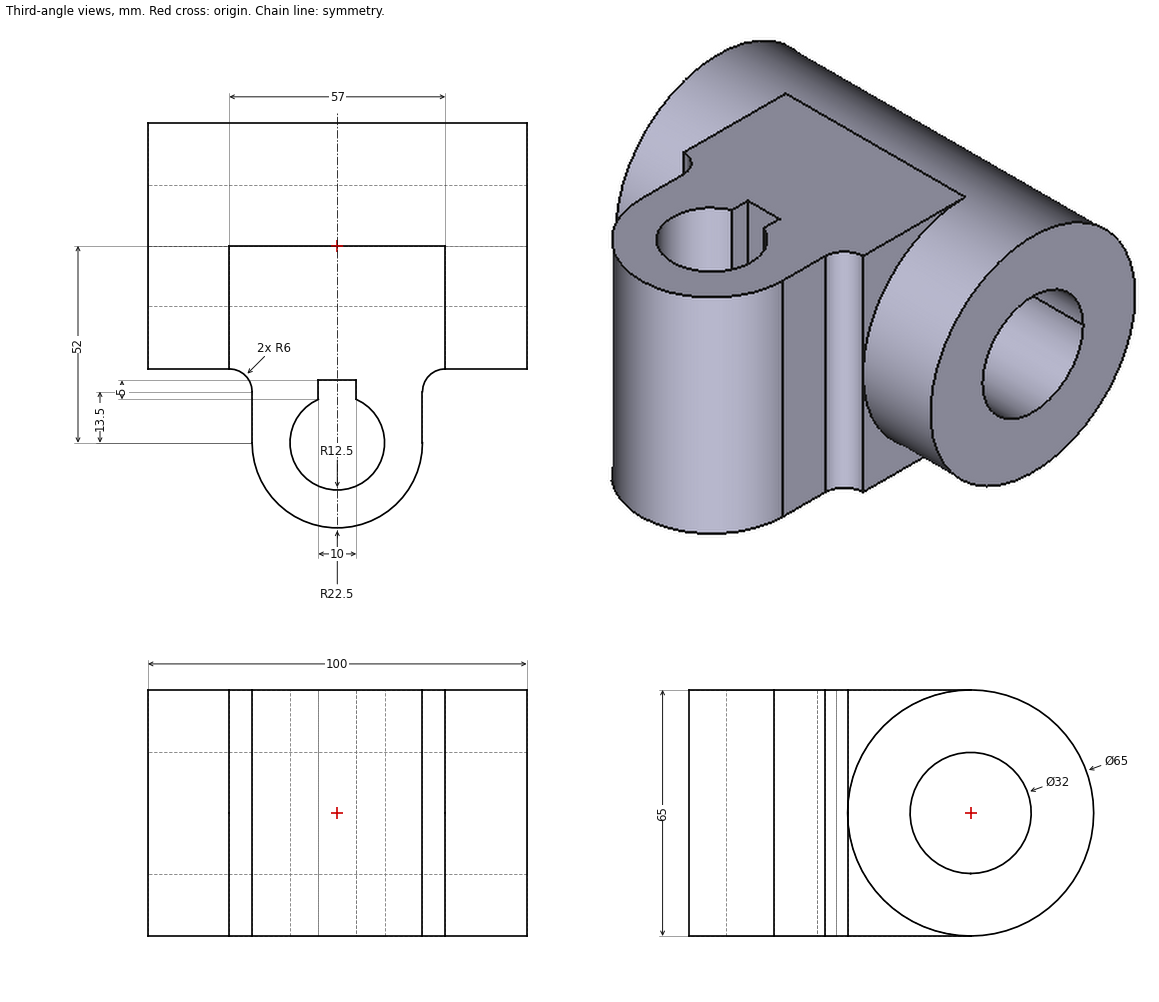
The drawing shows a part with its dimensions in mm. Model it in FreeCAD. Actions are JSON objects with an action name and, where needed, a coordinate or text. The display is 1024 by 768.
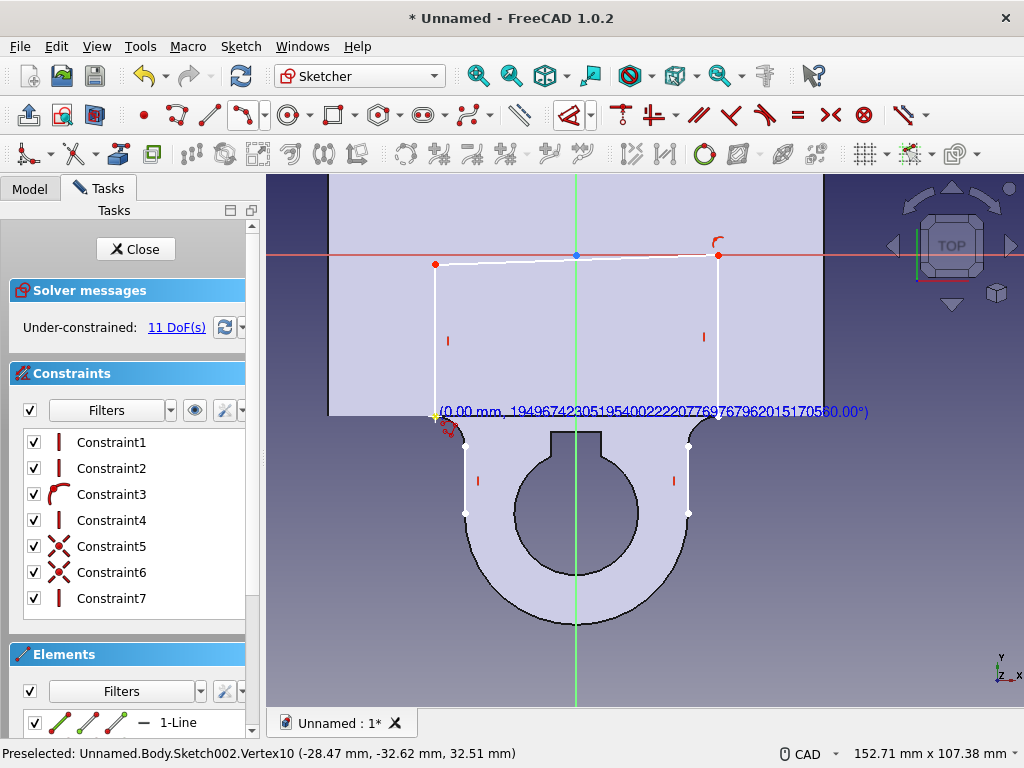
{"action": "left_click", "coordinate": [242, 116]}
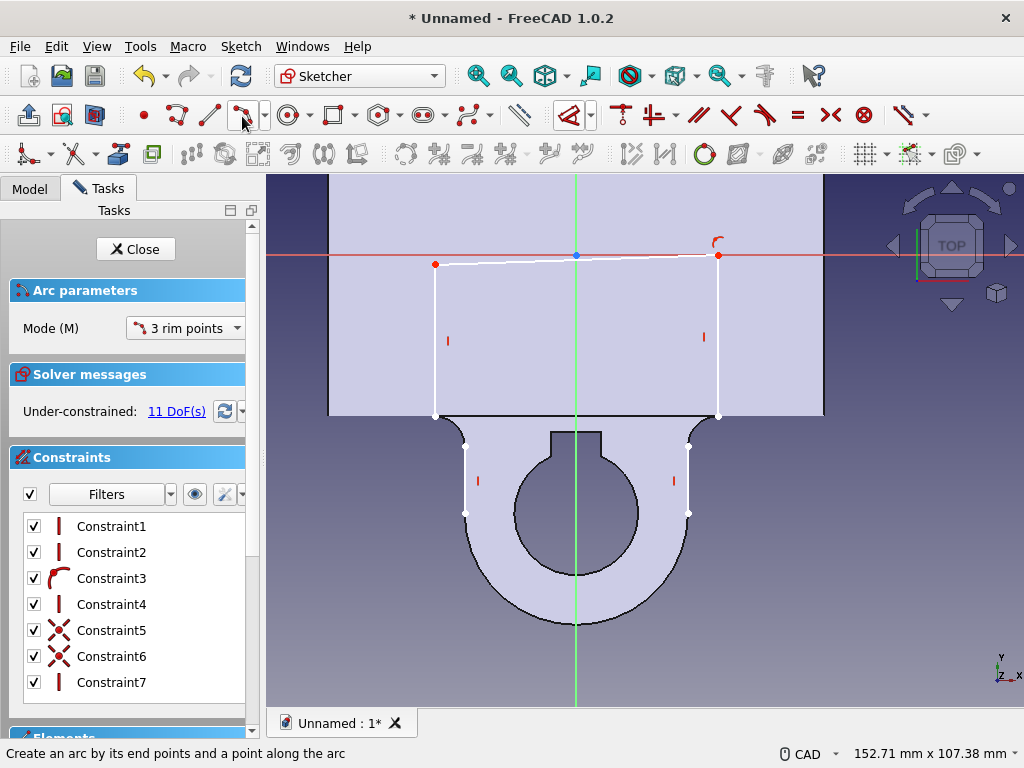
{"action": "left_click", "coordinate": [465, 514]}
{"action": "left_click", "coordinate": [688, 514]}
{"action": "left_click", "coordinate": [542, 619]}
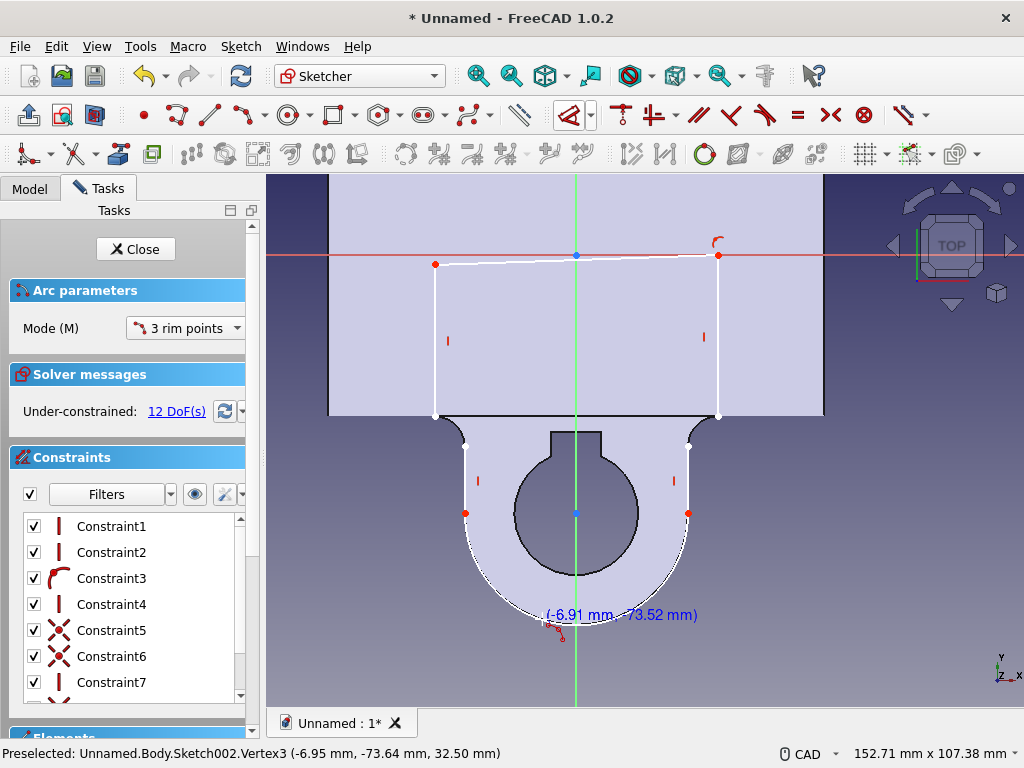
{"action": "left_click", "coordinate": [688, 447]}
{"action": "left_click", "coordinate": [718, 417]}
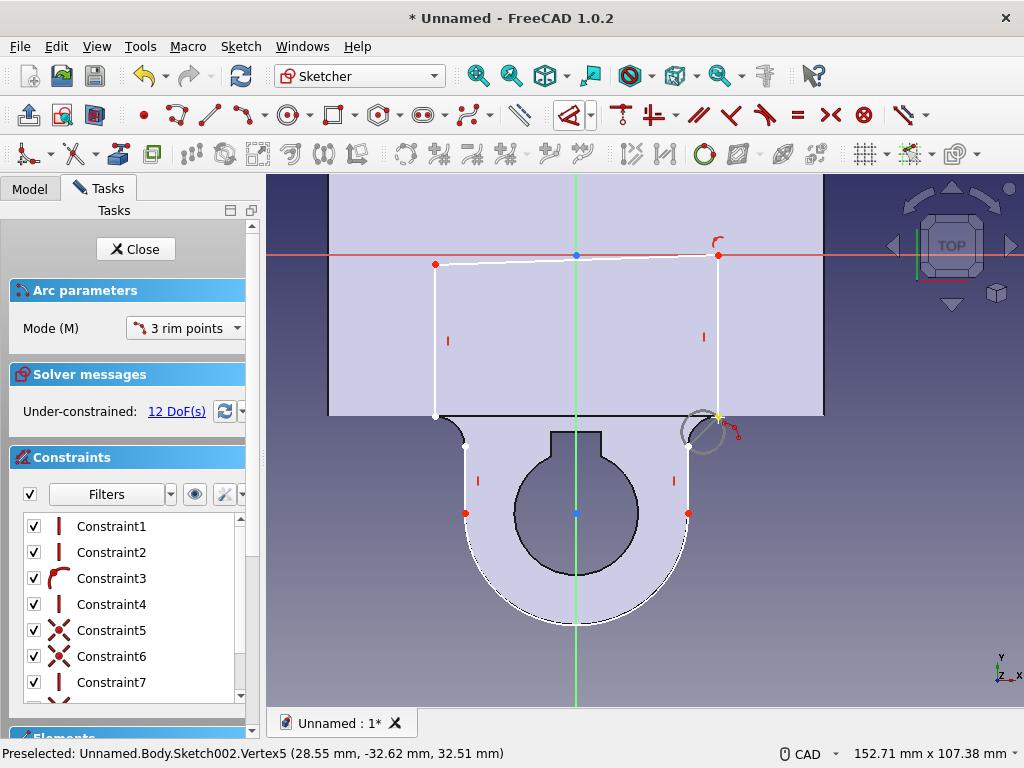
{"action": "scroll", "coordinate": [697, 425], "scroll_direction": "up", "scroll_amount": 3}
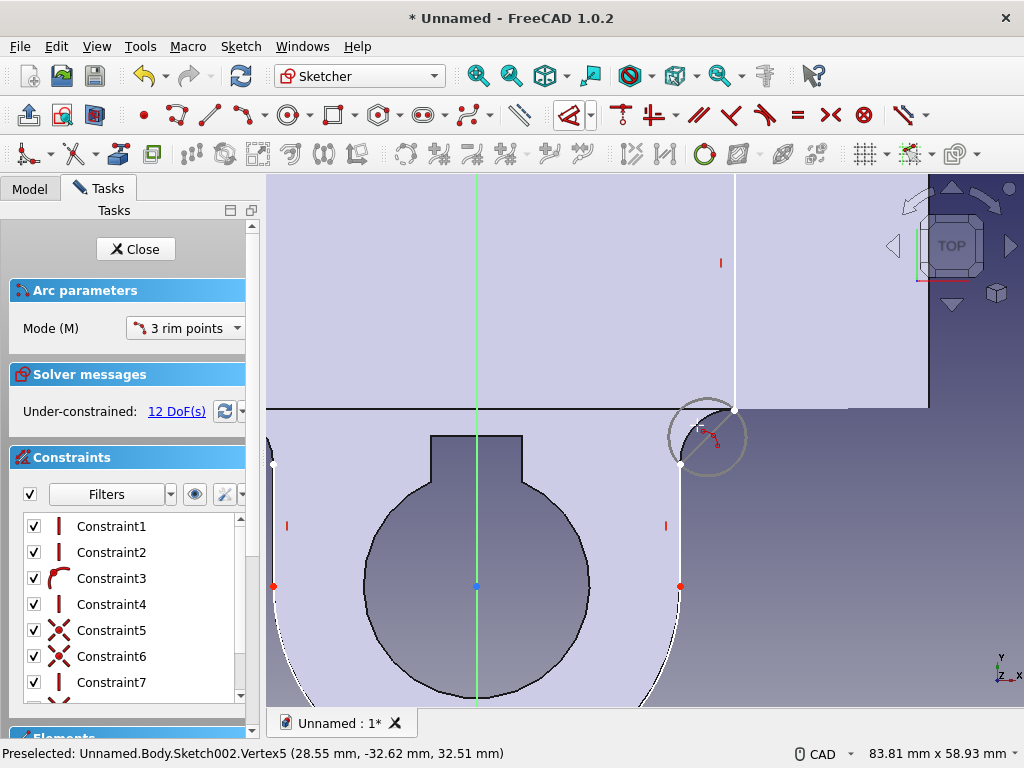
{"action": "left_click", "coordinate": [696, 425]}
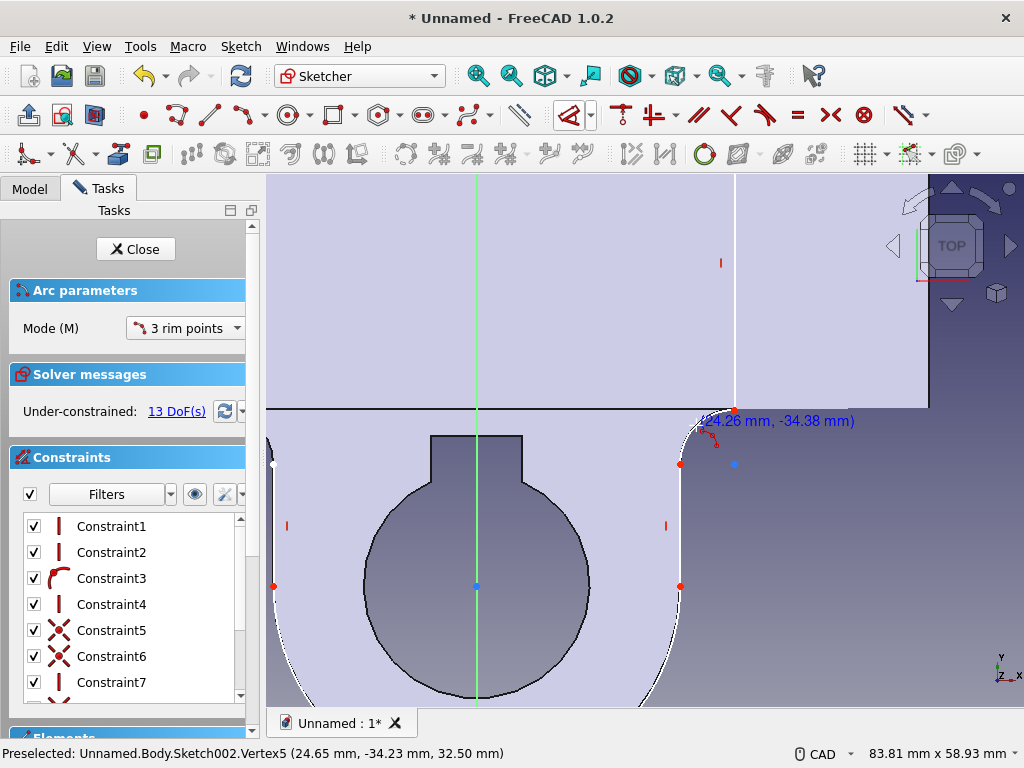
{"action": "scroll", "coordinate": [698, 427], "scroll_direction": "down", "scroll_amount": 3}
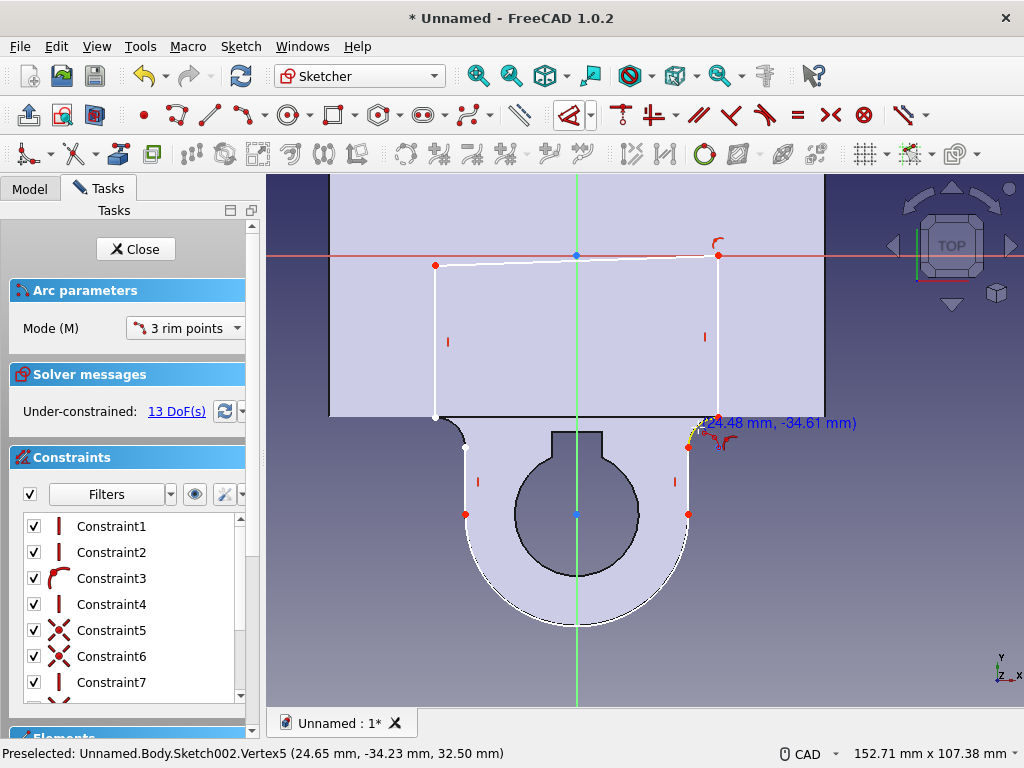
{"action": "left_click", "coordinate": [435, 418]}
{"action": "left_click", "coordinate": [465, 448]}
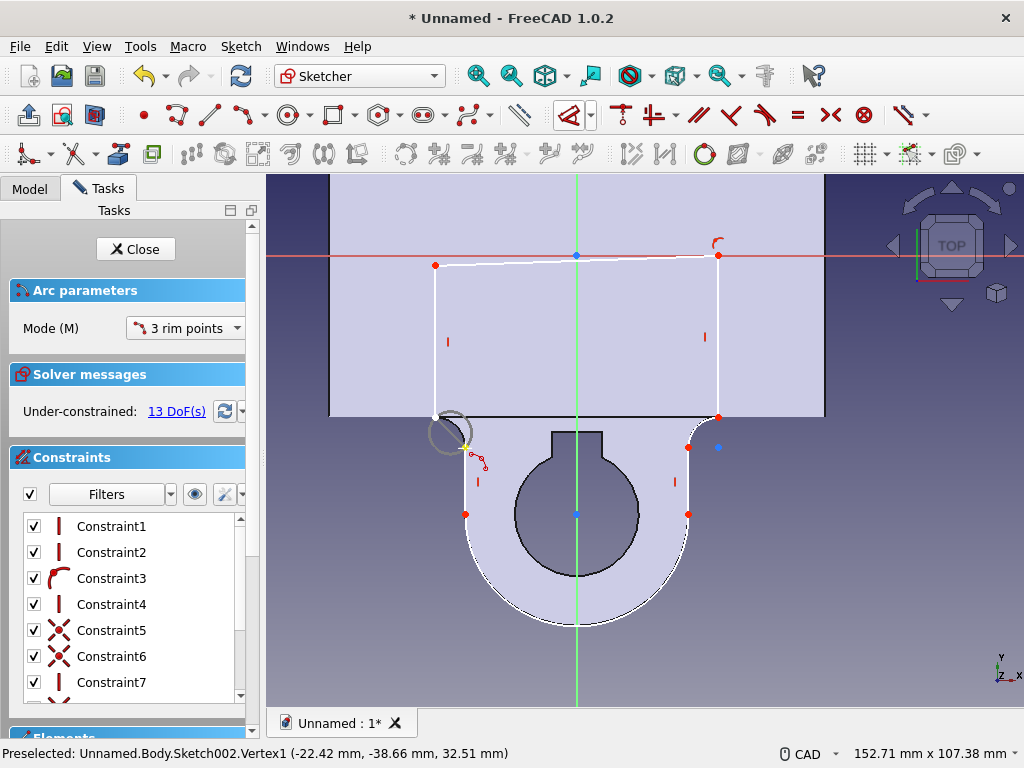
{"action": "scroll", "coordinate": [456, 426], "scroll_direction": "up", "scroll_amount": 3}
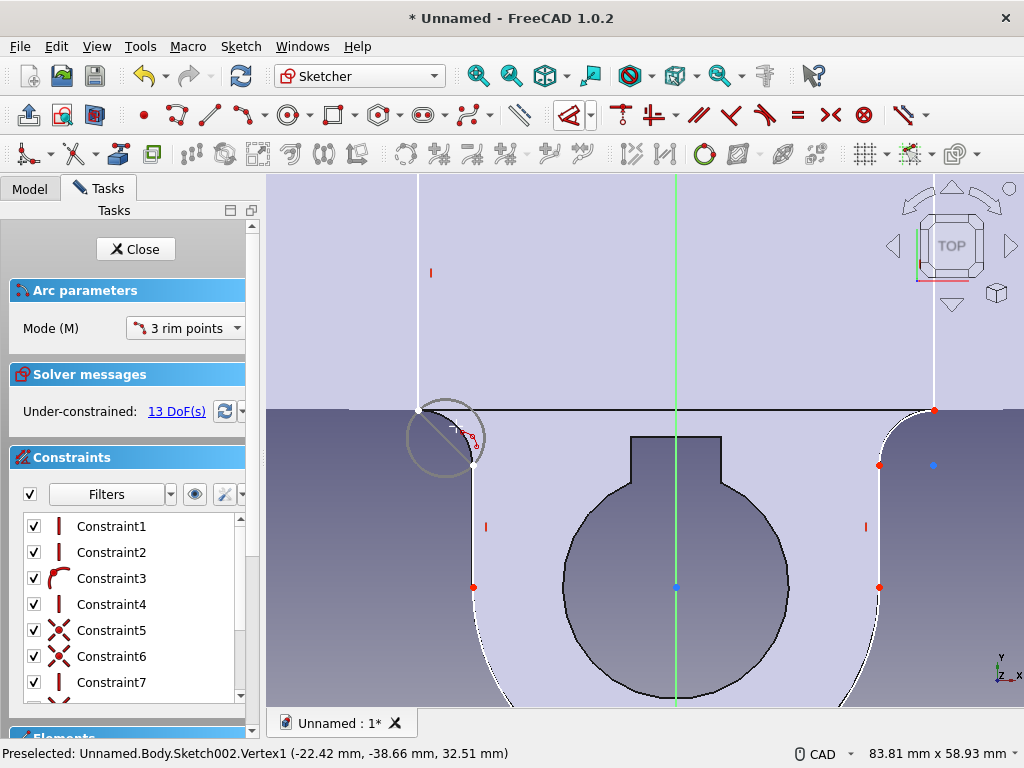
{"action": "left_click", "coordinate": [456, 426]}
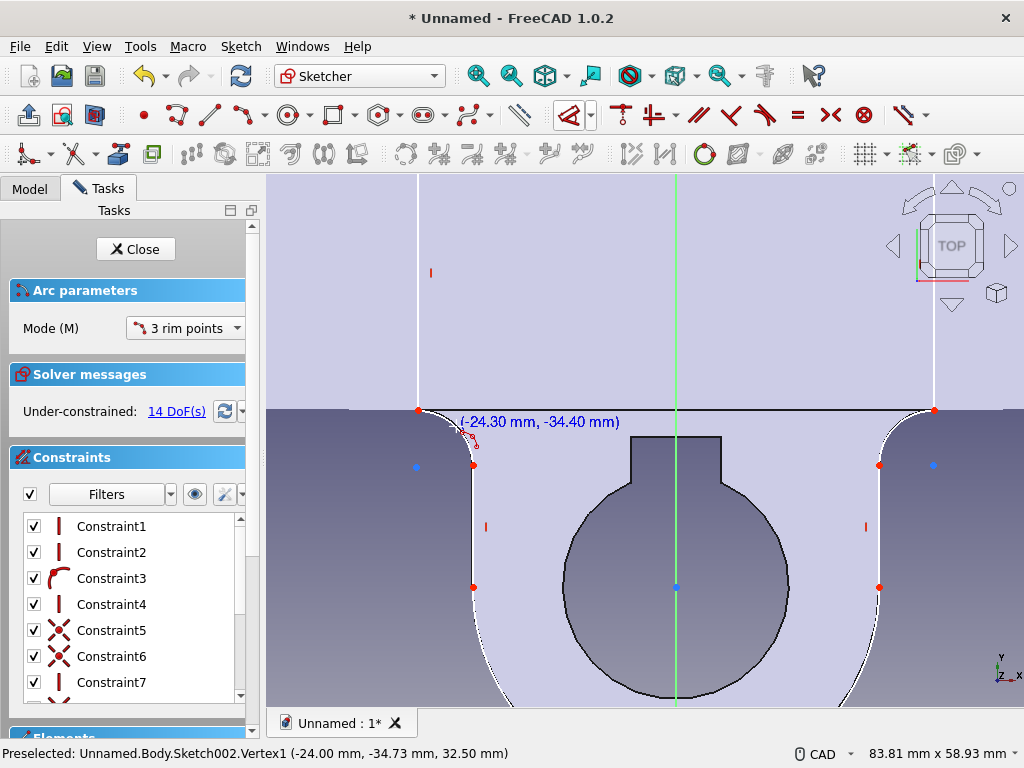
{"action": "left_click", "coordinate": [177, 116]}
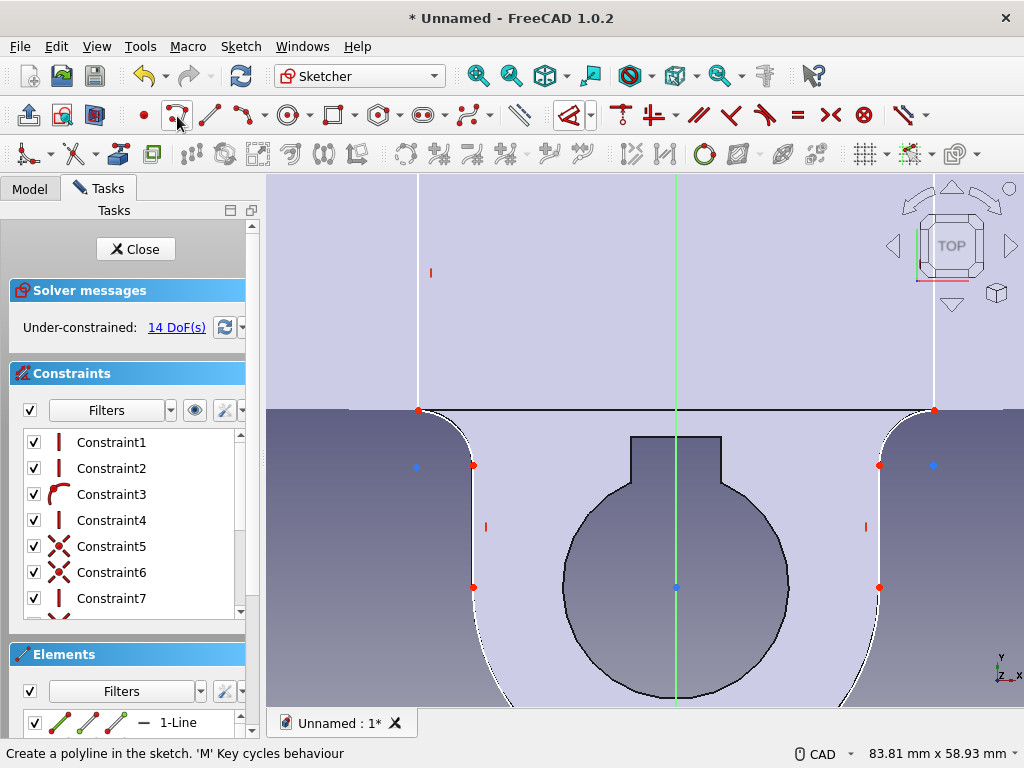
{"action": "left_click", "coordinate": [631, 483]}
{"action": "left_click", "coordinate": [631, 437]}
{"action": "left_click", "coordinate": [721, 437]}
{"action": "left_click", "coordinate": [721, 483]}
{"action": "right_click", "coordinate": [721, 483]}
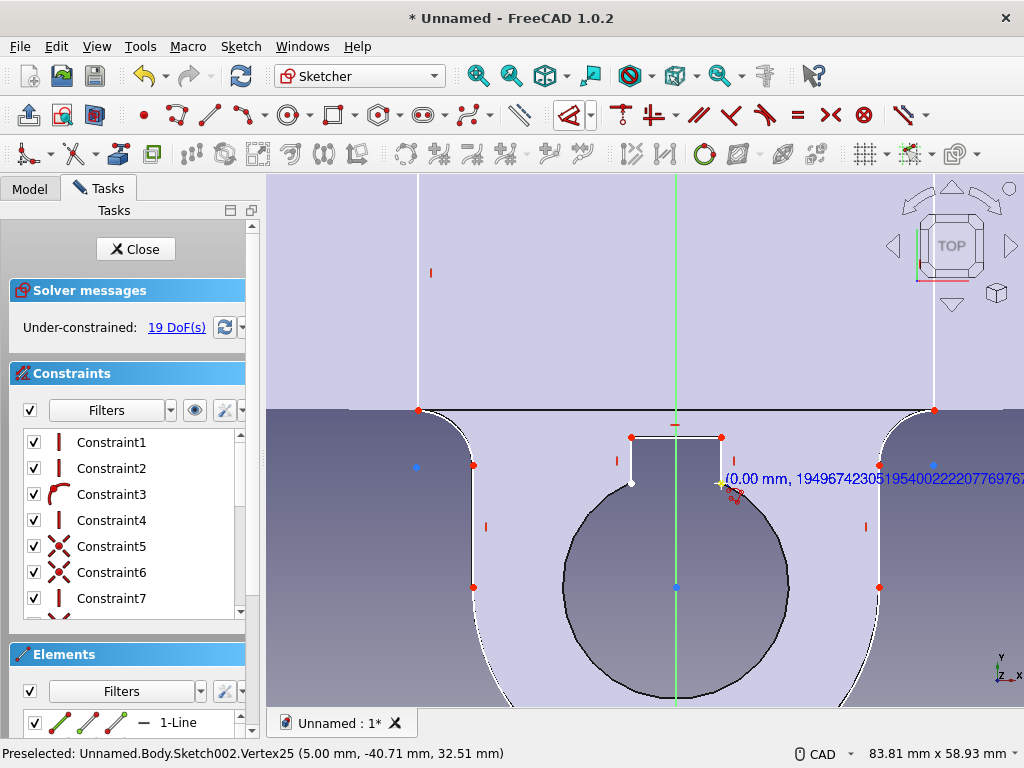
{"action": "key", "text": "g 3 a"}